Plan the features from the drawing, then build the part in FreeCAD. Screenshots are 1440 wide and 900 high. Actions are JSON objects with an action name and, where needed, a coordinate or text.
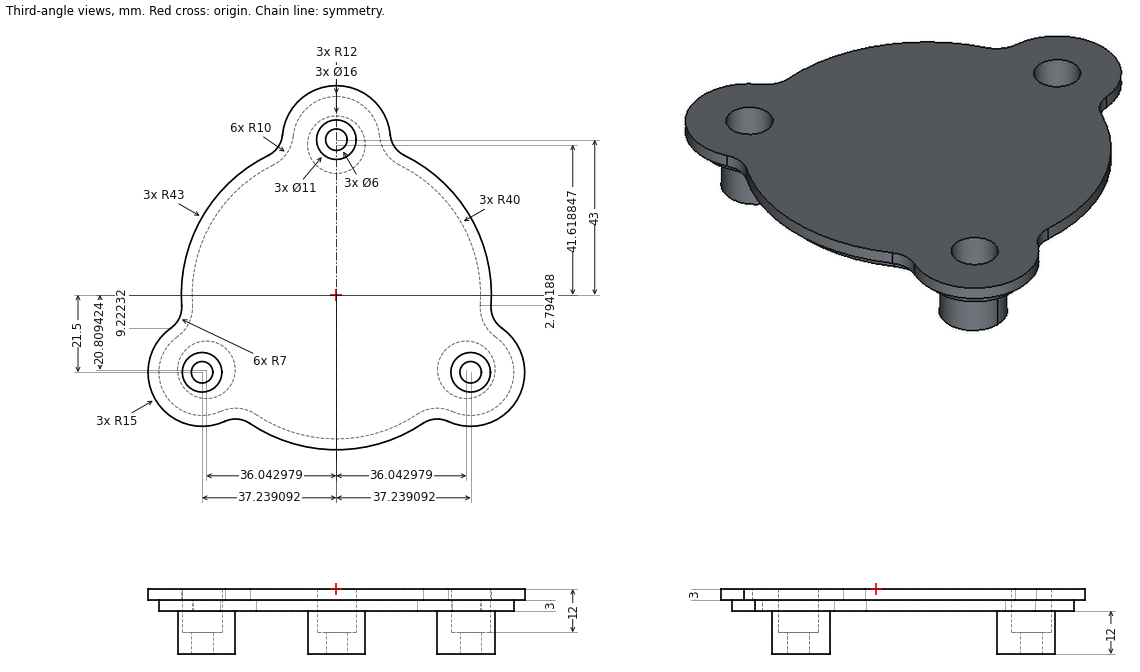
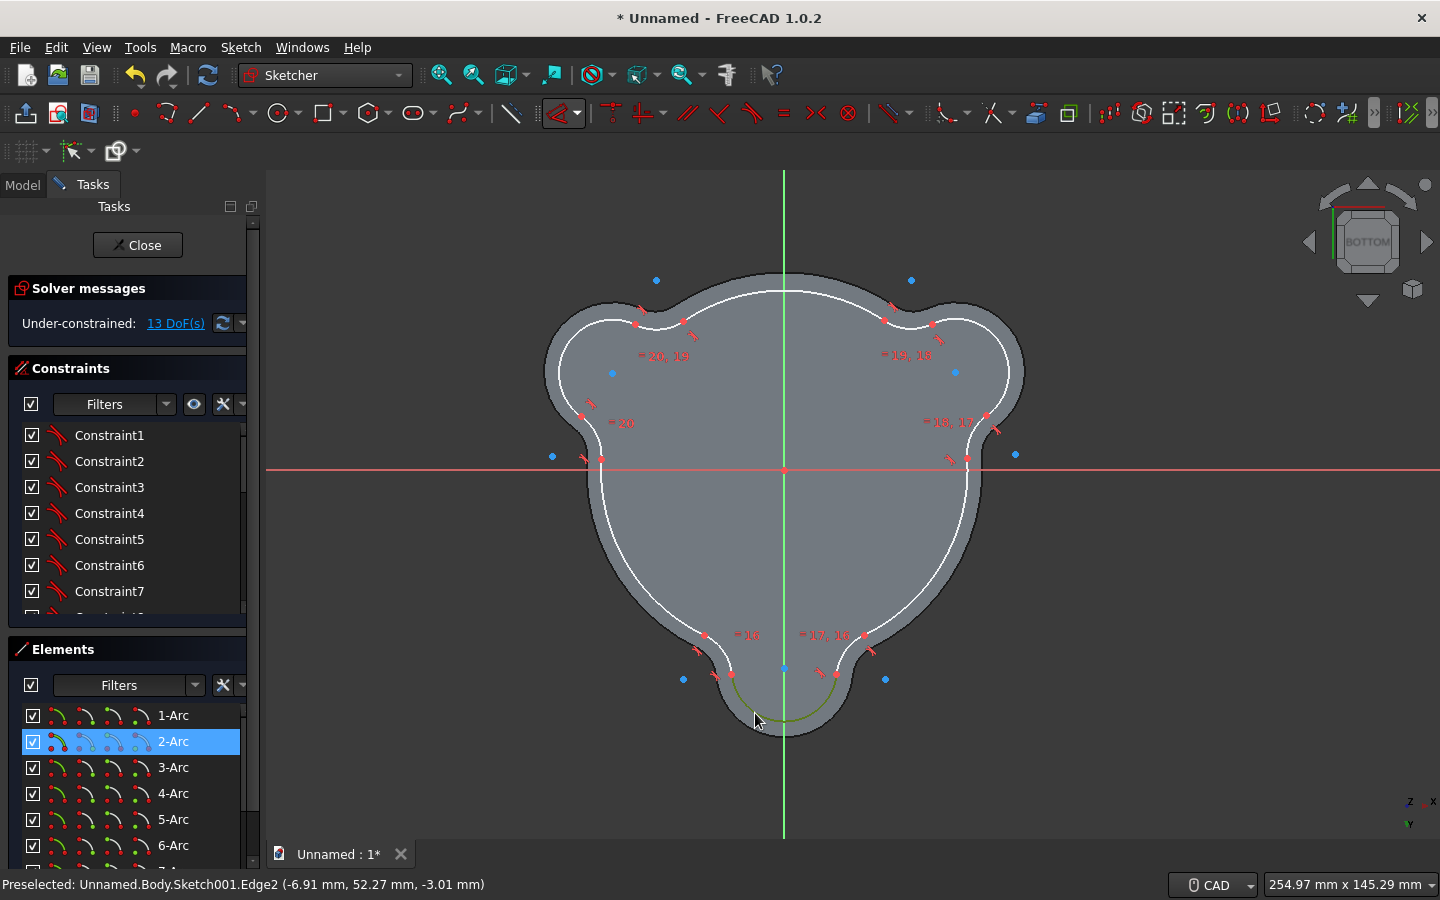
{"action": "left_click", "coordinate": [1009, 375]}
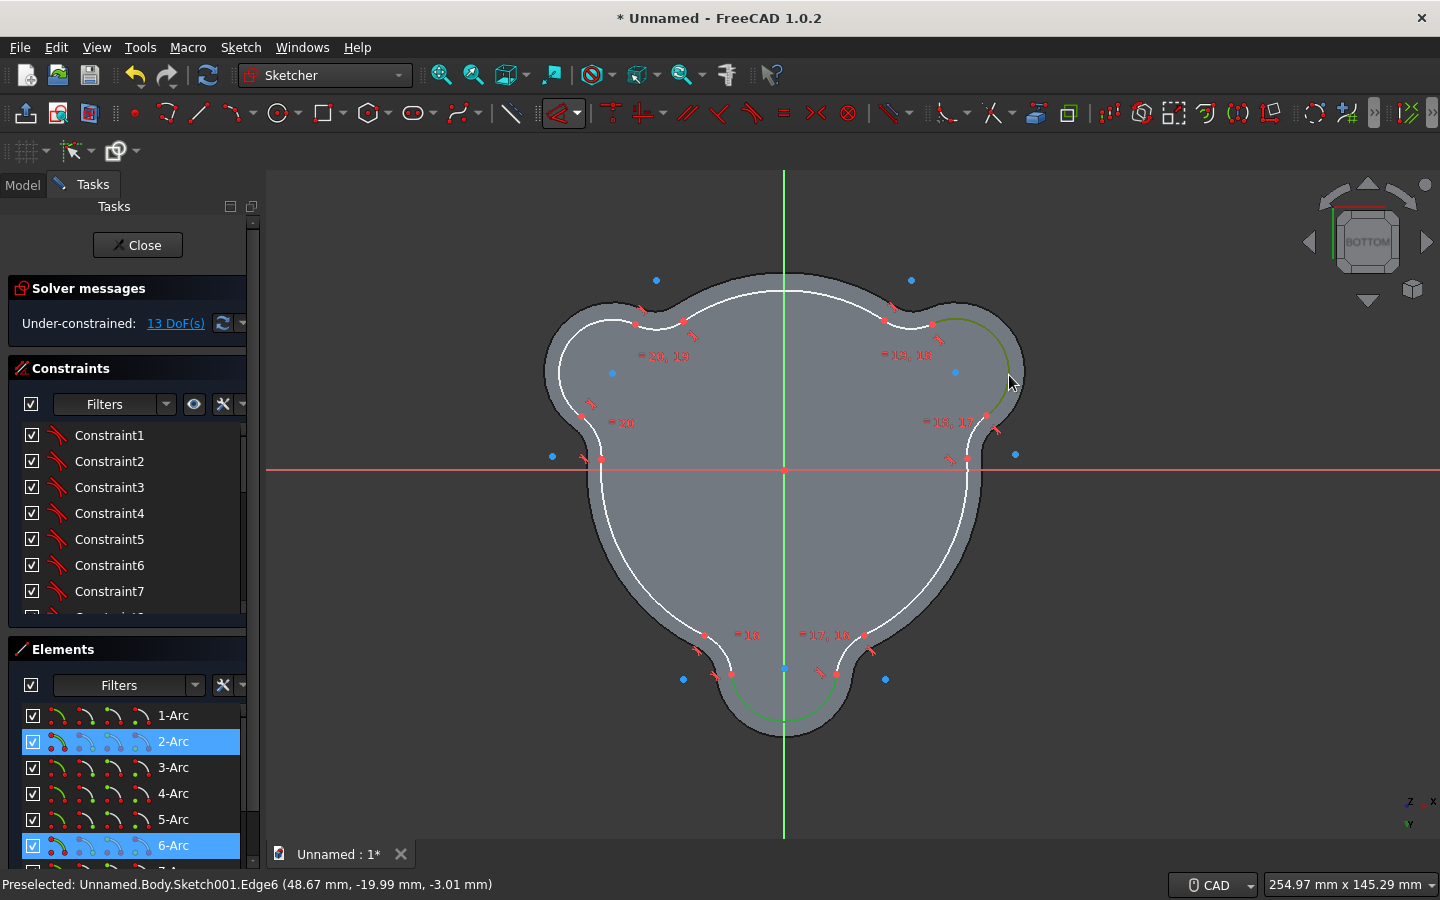
{"action": "left_click", "coordinate": [590, 325]}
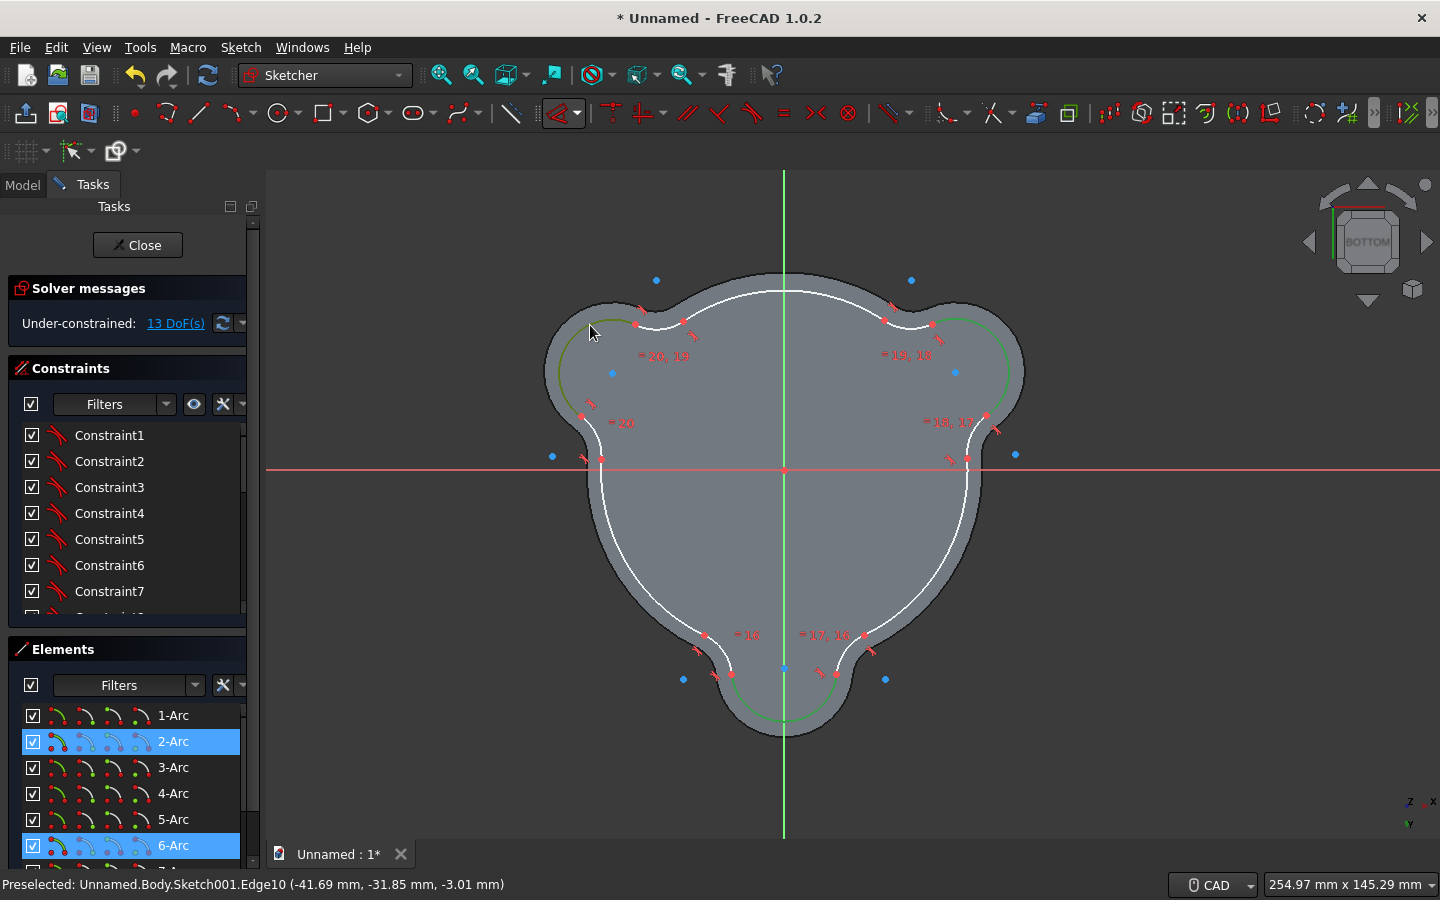
{"action": "left_click", "coordinate": [784, 114]}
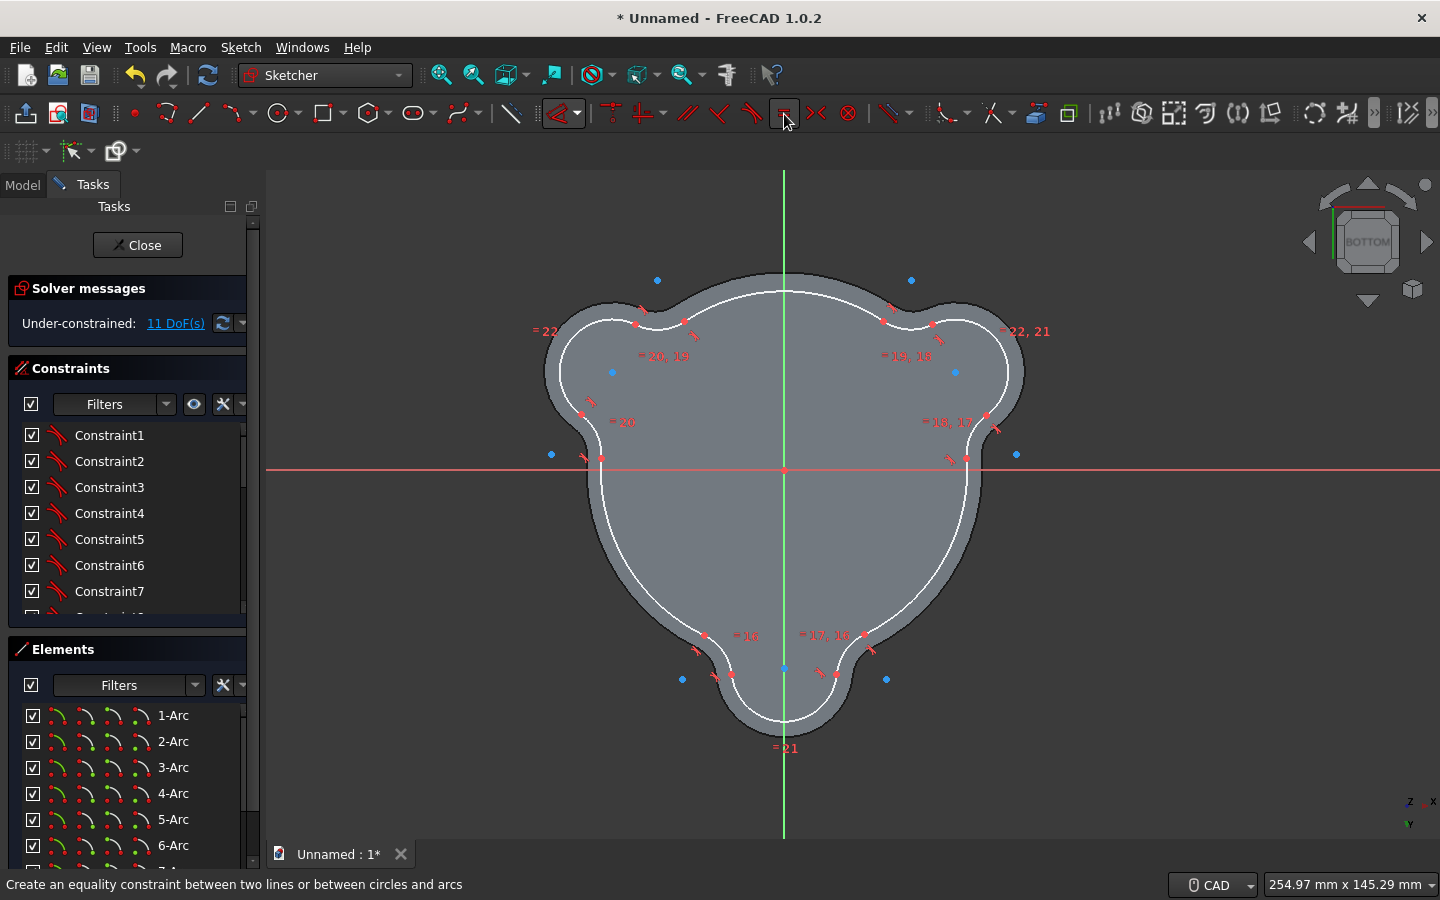
{"action": "left_click", "coordinate": [917, 596]}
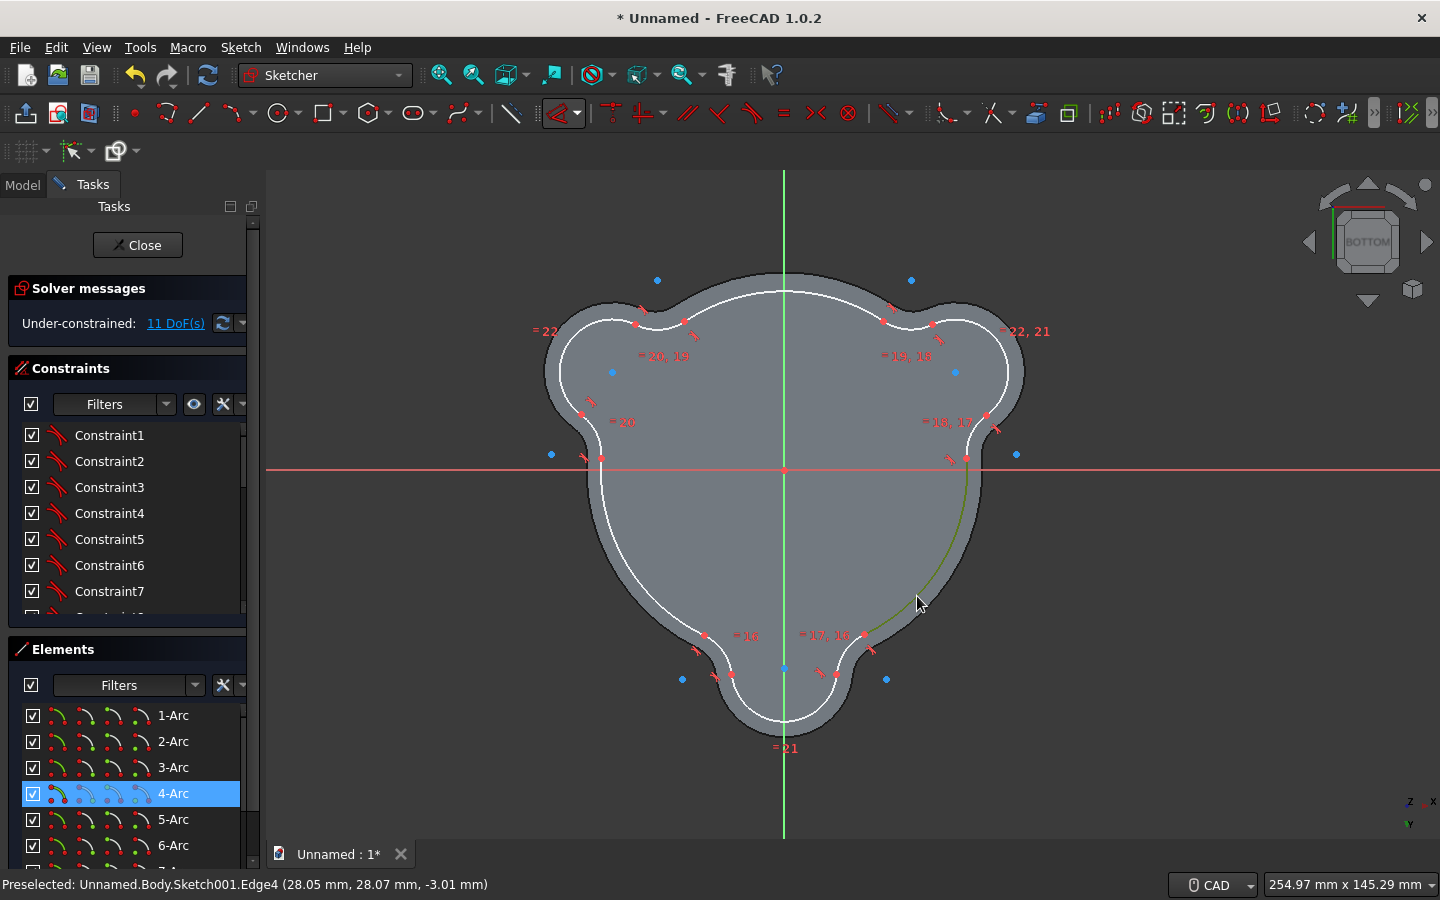
{"action": "left_click", "coordinate": [826, 296]}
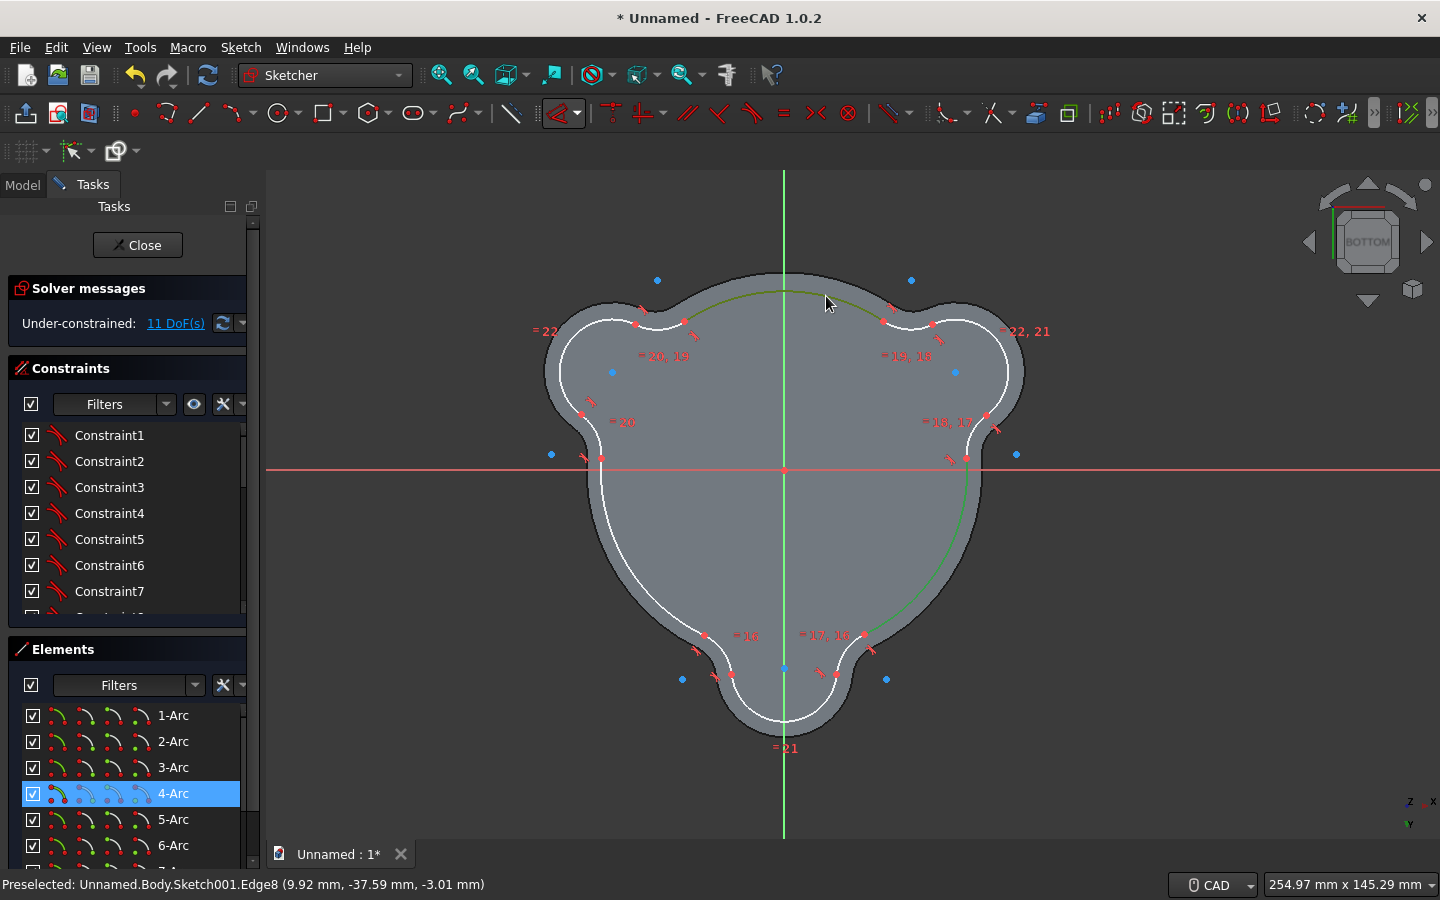
{"action": "left_click", "coordinate": [608, 523]}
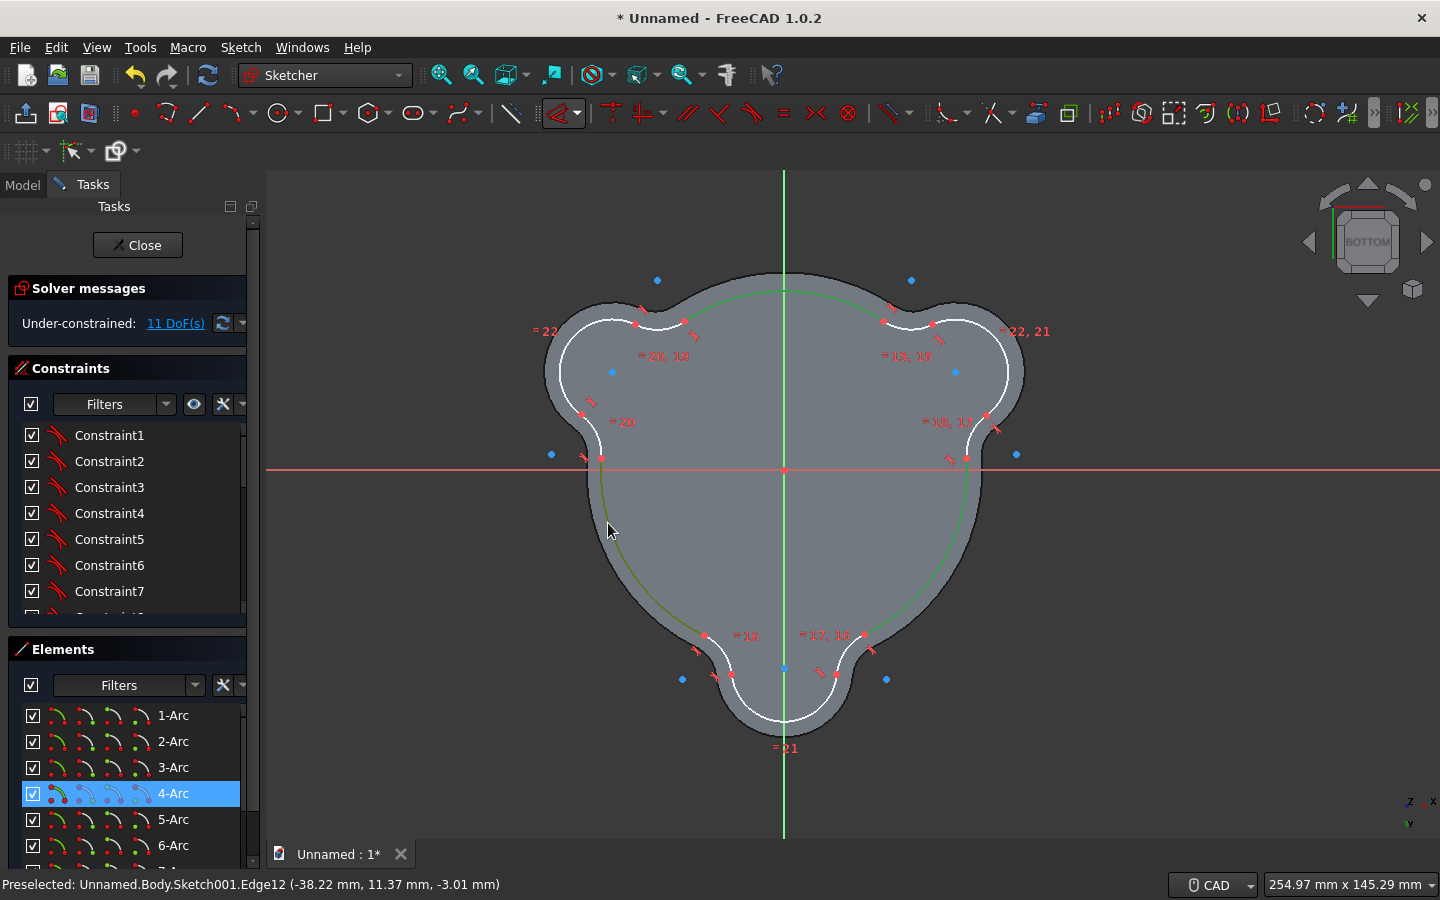
{"action": "left_click", "coordinate": [784, 114]}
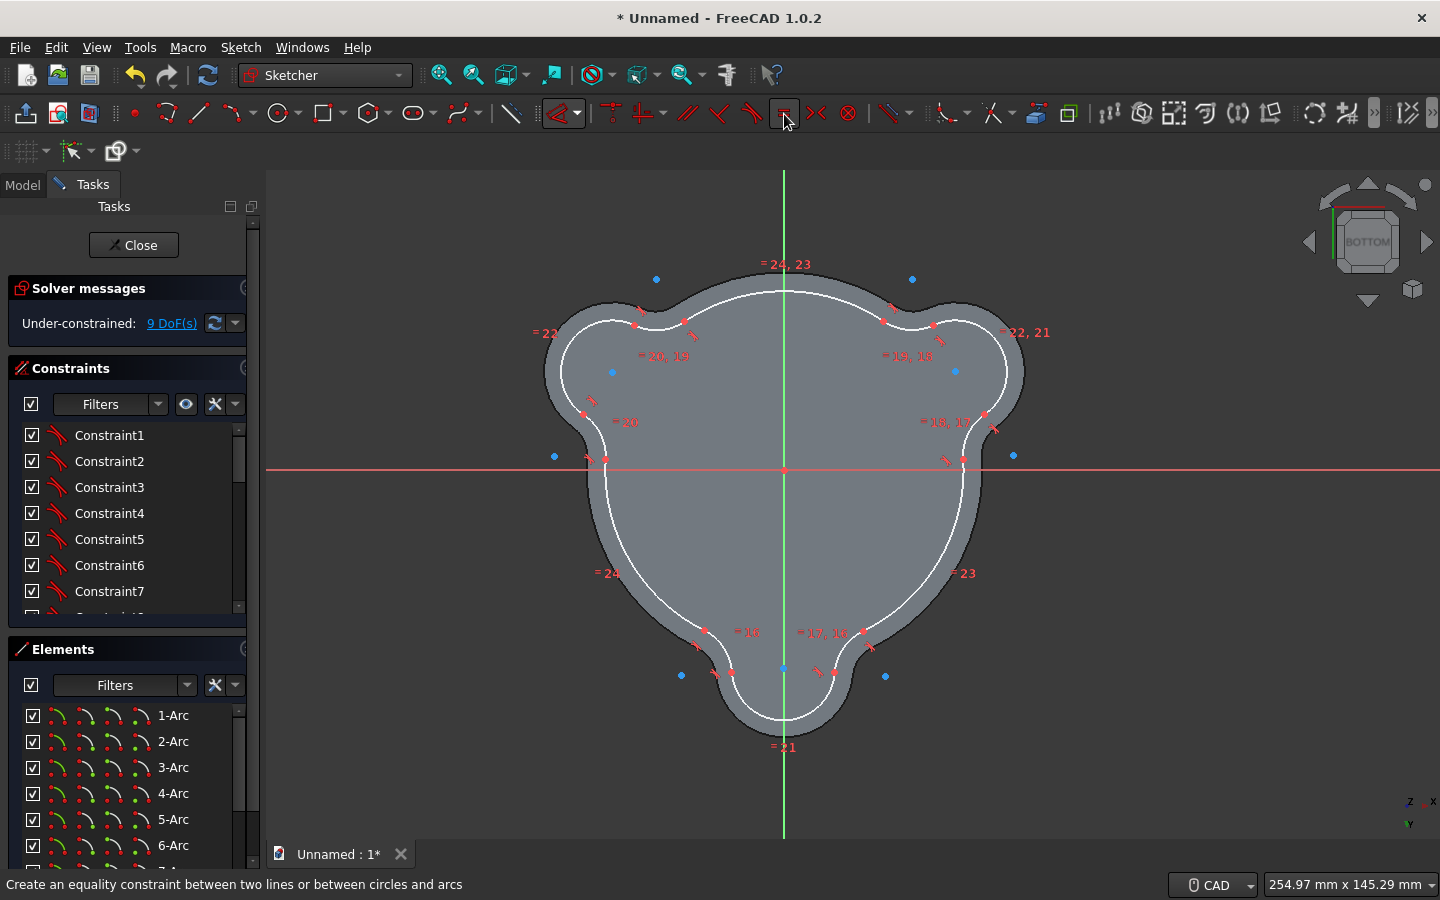
{"action": "left_click", "coordinate": [783, 669]}